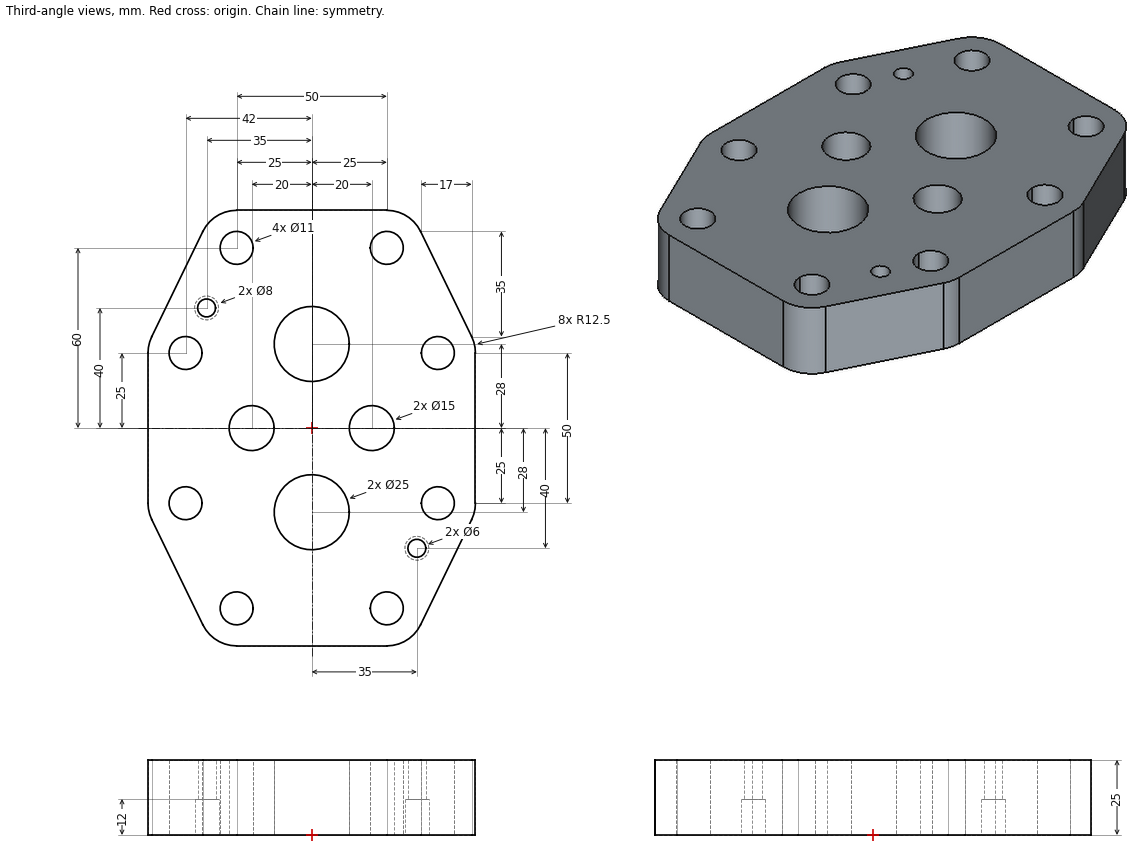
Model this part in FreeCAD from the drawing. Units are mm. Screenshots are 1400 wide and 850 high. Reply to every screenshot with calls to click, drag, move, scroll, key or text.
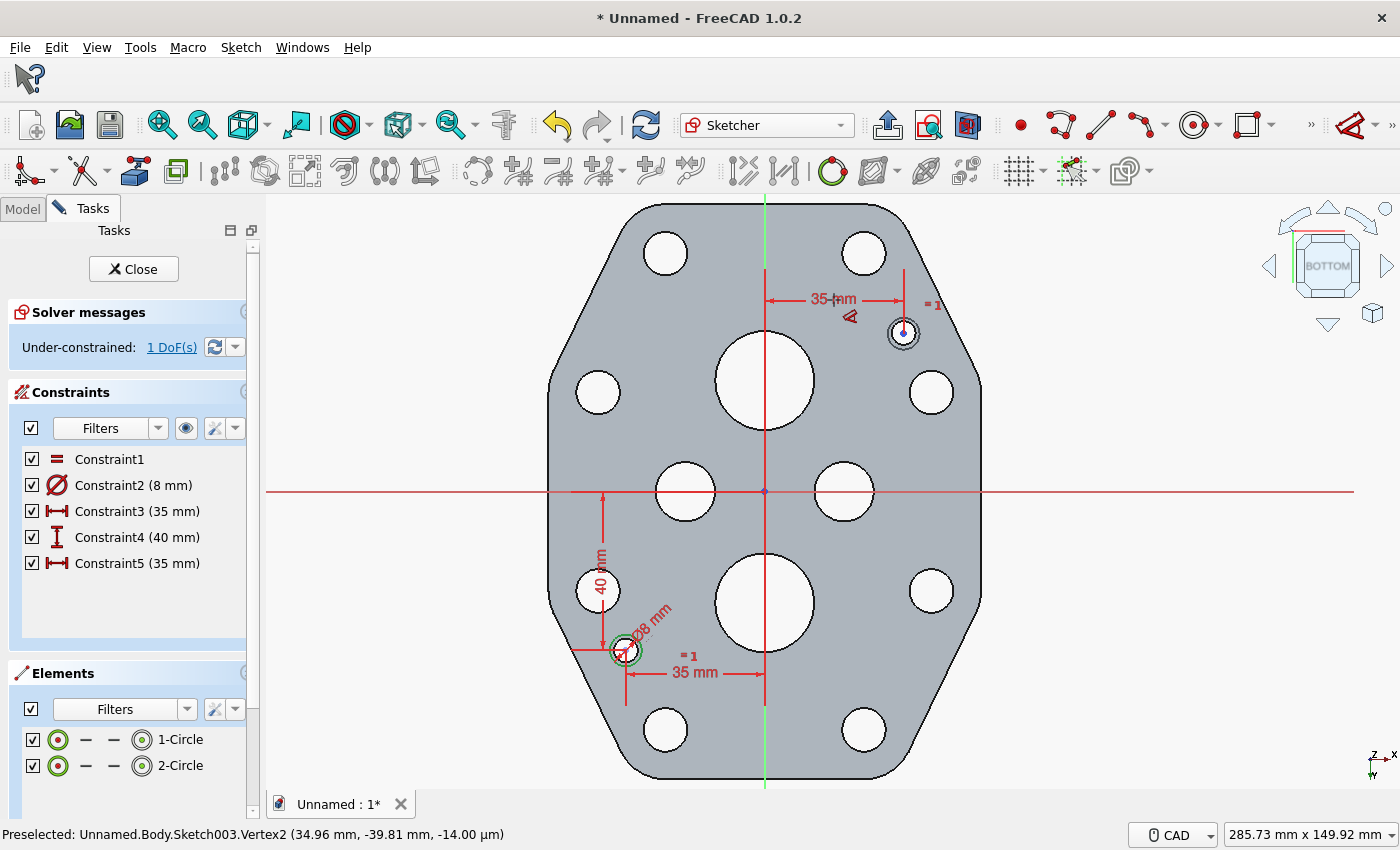
click(904, 334)
click(938, 413)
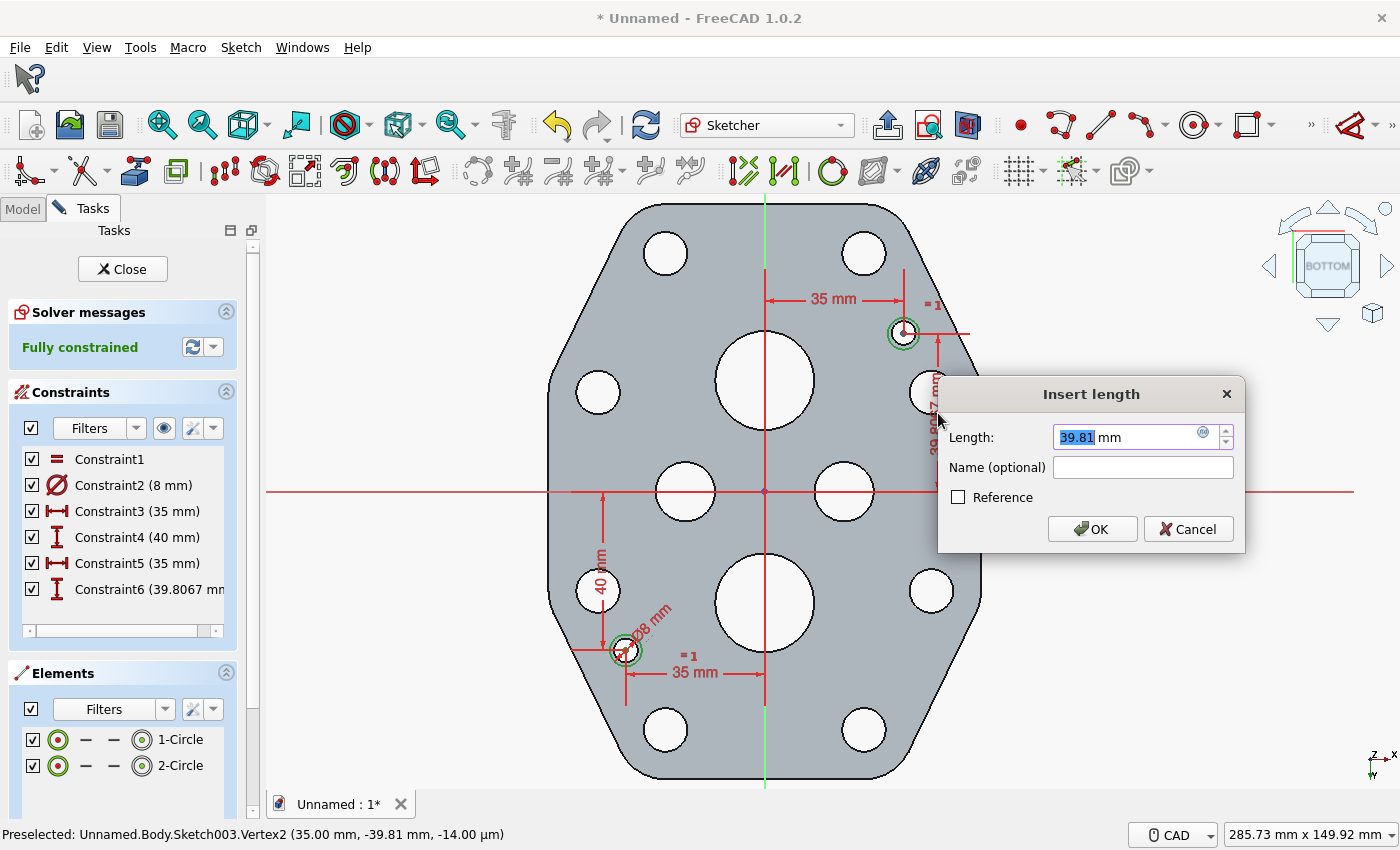
text(40)
key(Return)
key(Escape)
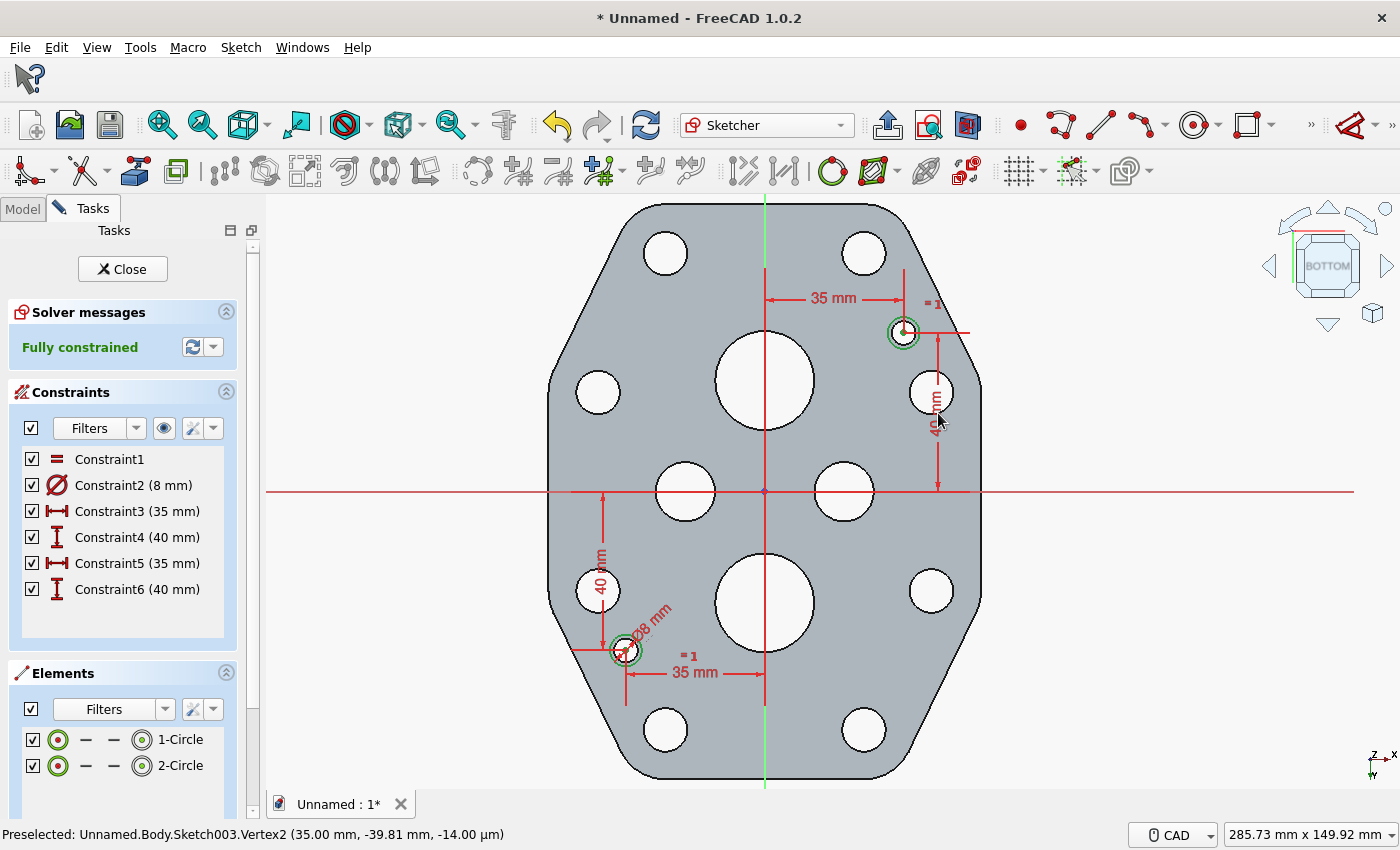
click(123, 269)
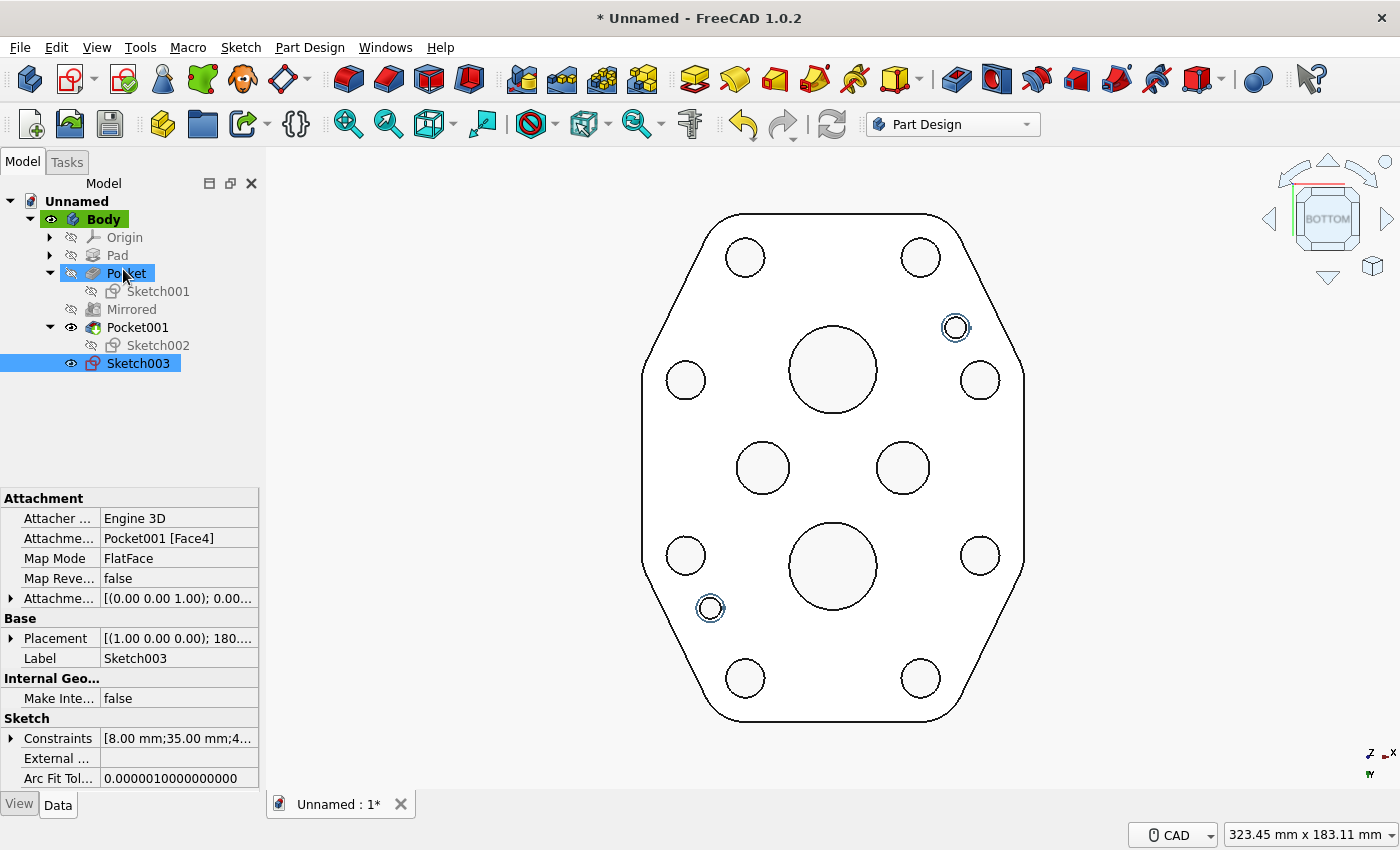
click(958, 80)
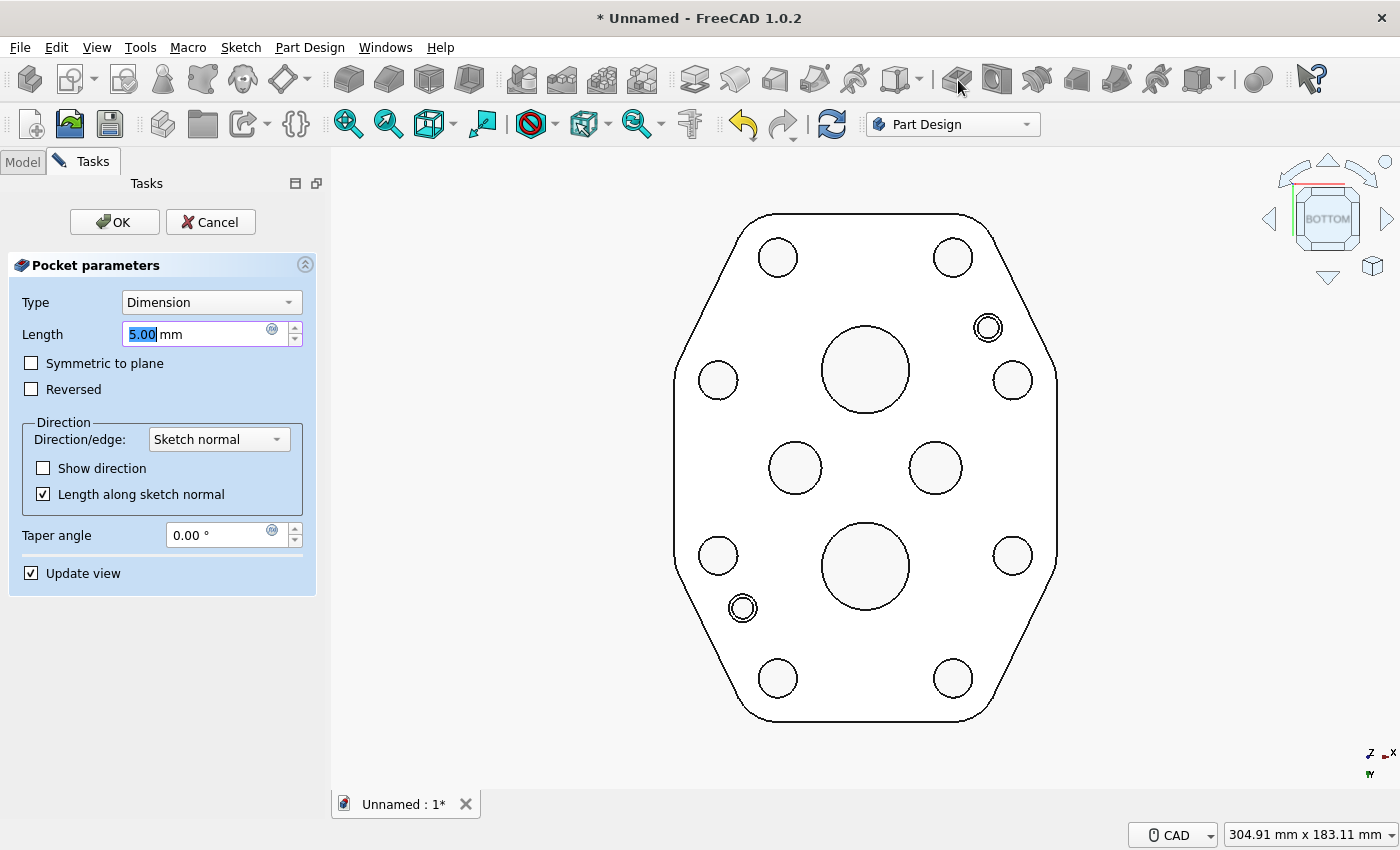
text(12)
key(Tab)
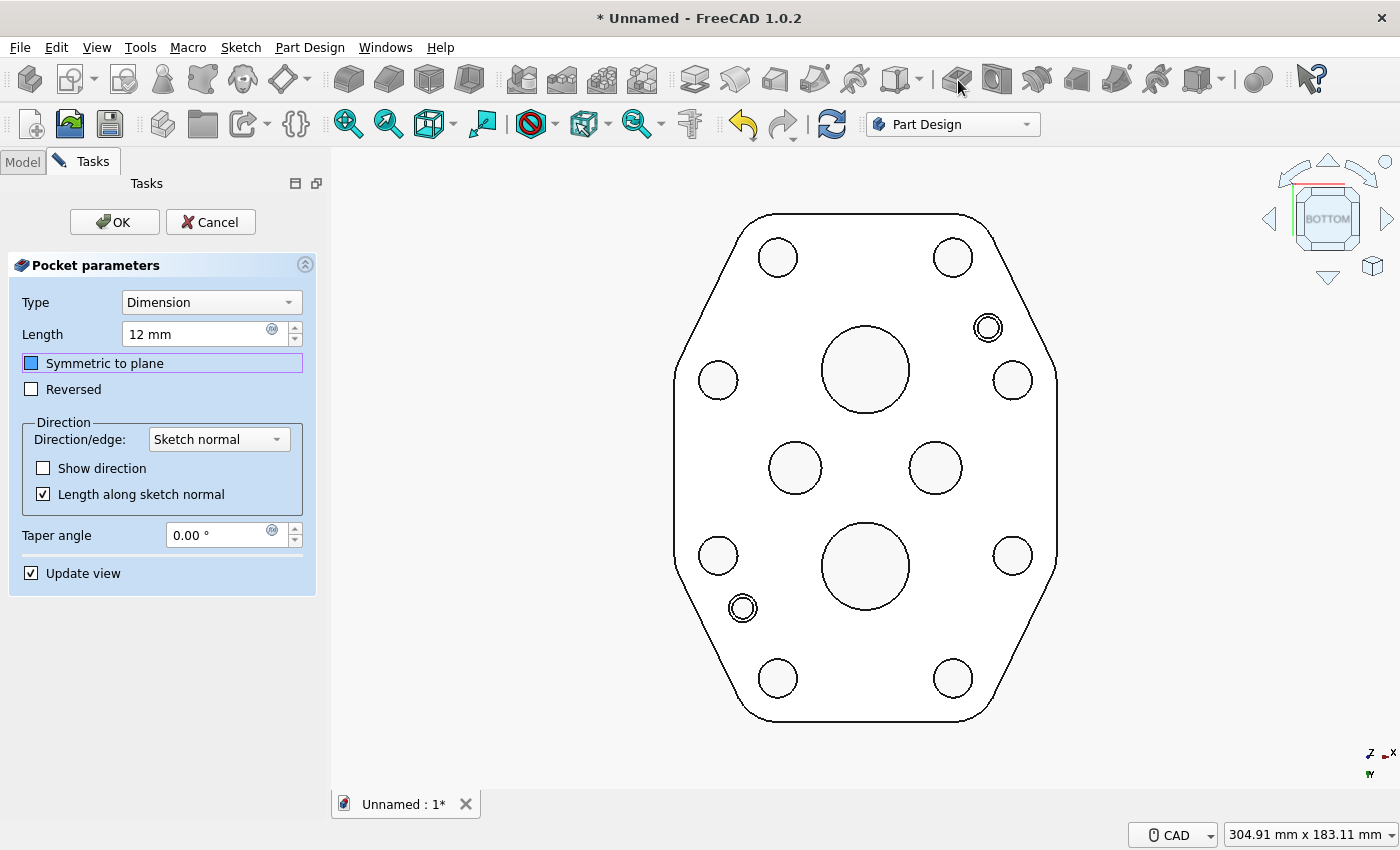
click(115, 222)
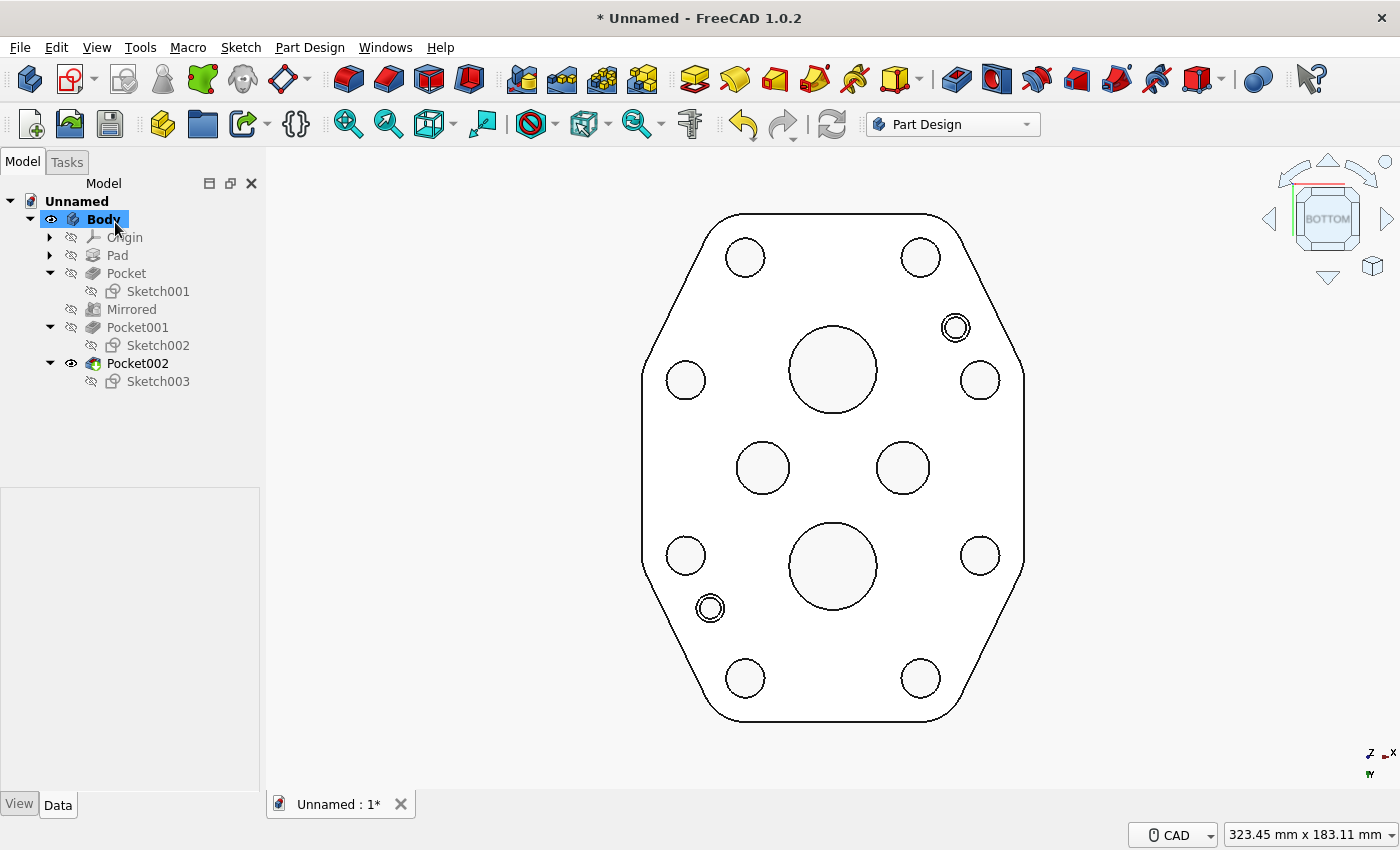
key(0)